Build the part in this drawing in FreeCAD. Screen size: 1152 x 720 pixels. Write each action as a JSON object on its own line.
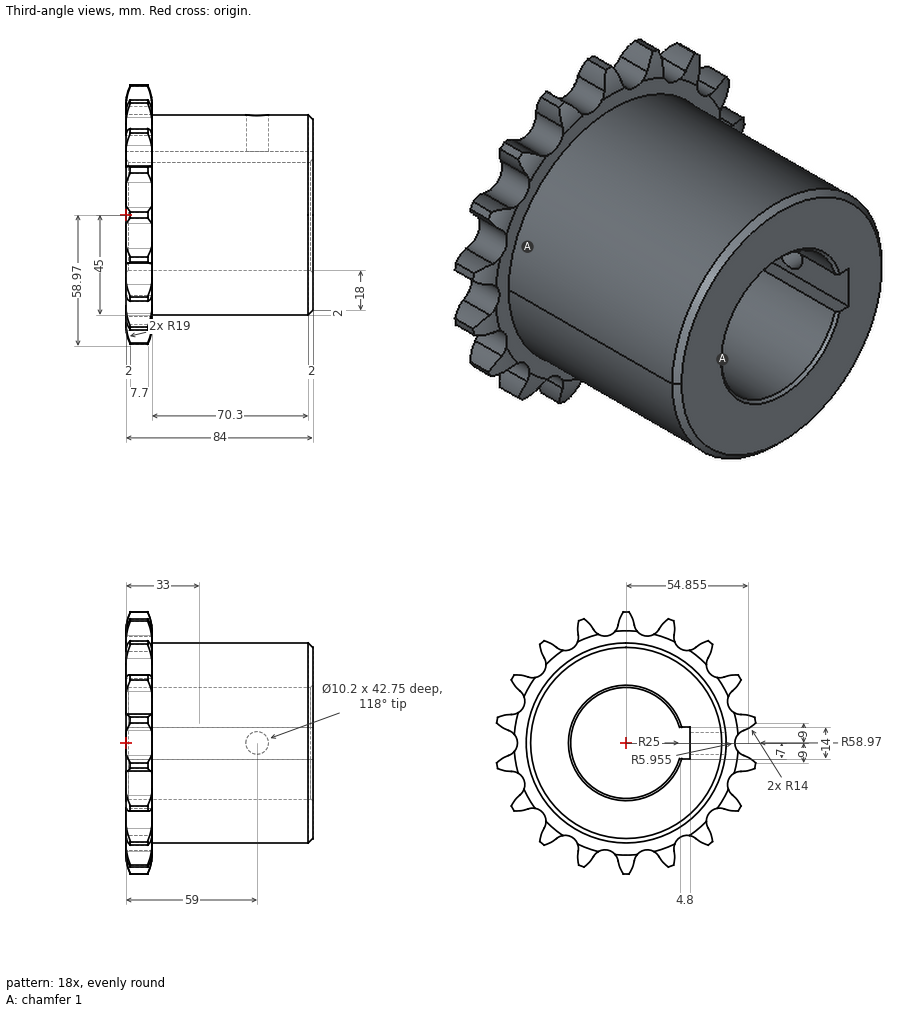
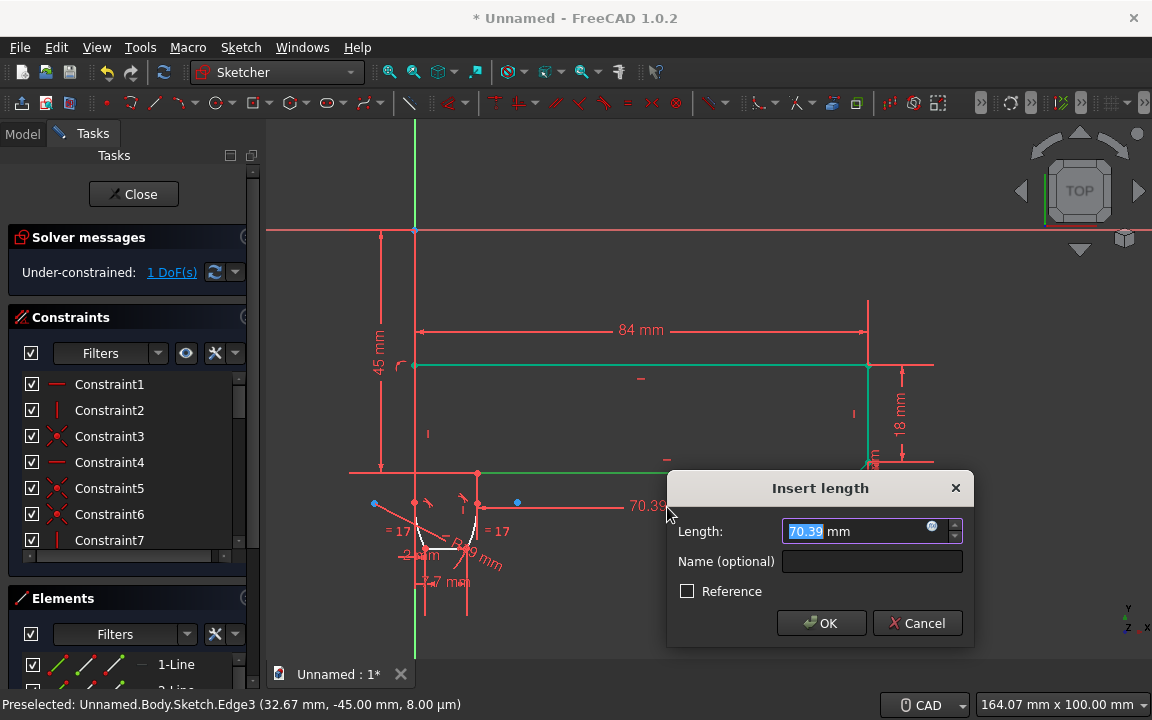
{"action": "type", "text": "70.3"}
{"action": "key", "text": "Return"}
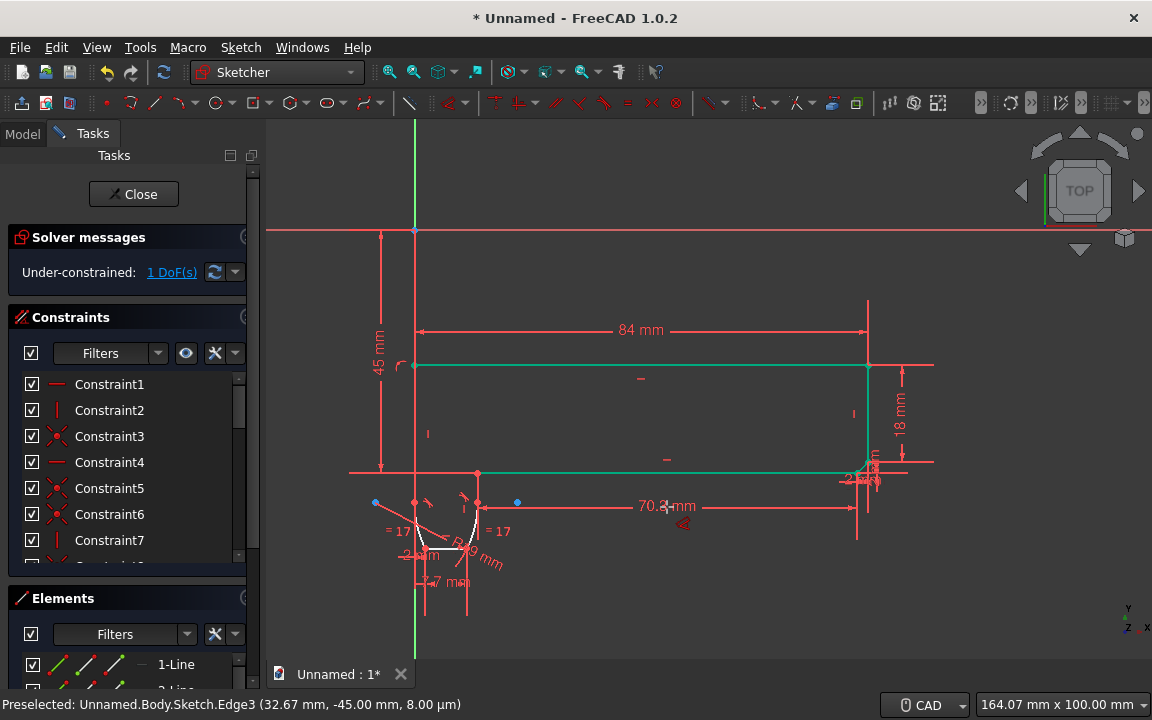
{"action": "left_click", "coordinate": [425, 549]}
{"action": "left_click", "coordinate": [381, 389]}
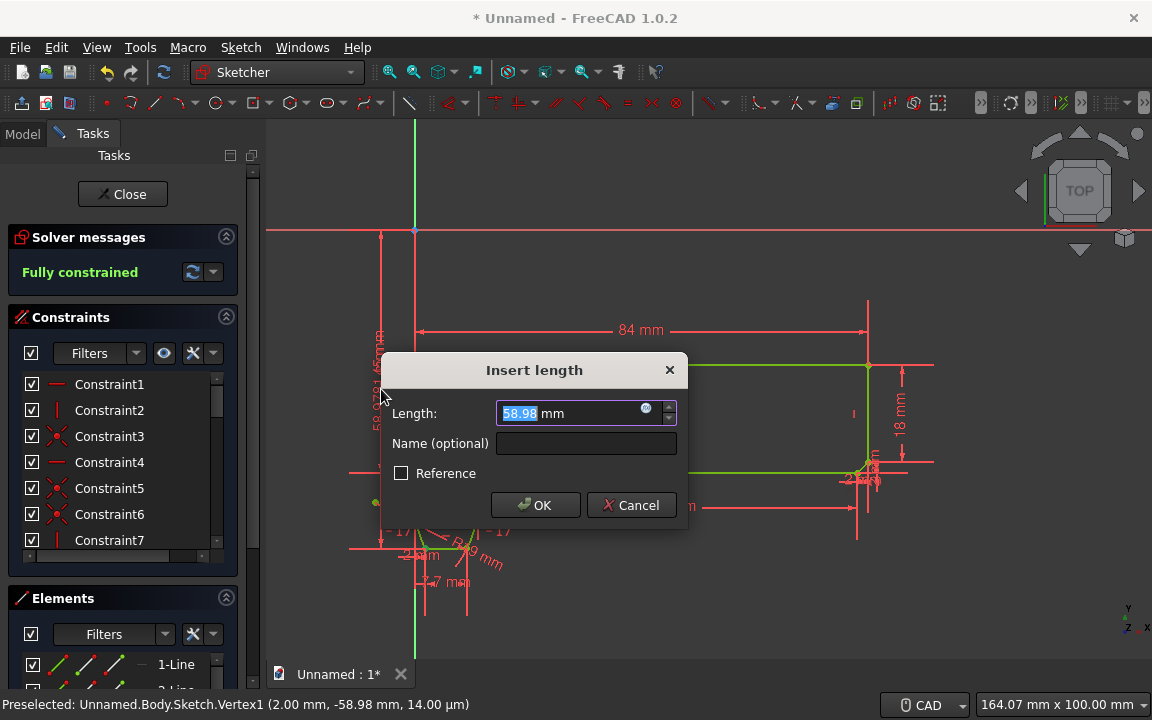
{"action": "type", "text": "58.97"}
{"action": "key", "text": "Return"}
{"action": "key", "text": "Escape"}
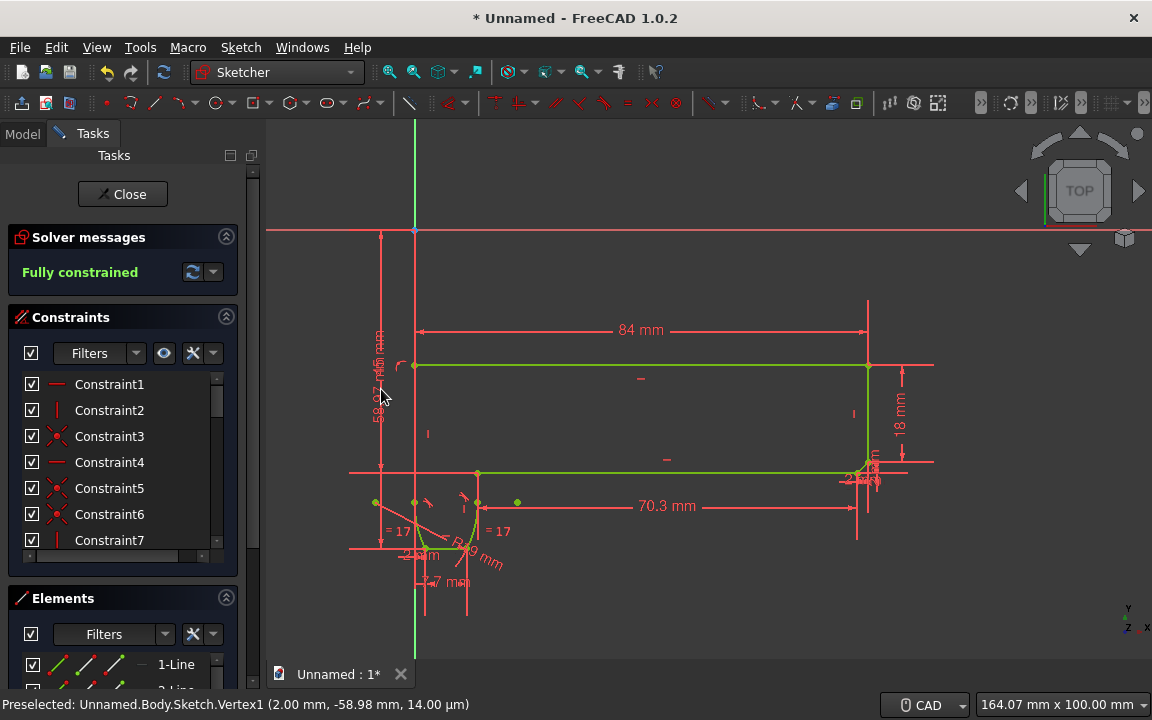
{"action": "left_click", "coordinate": [123, 194]}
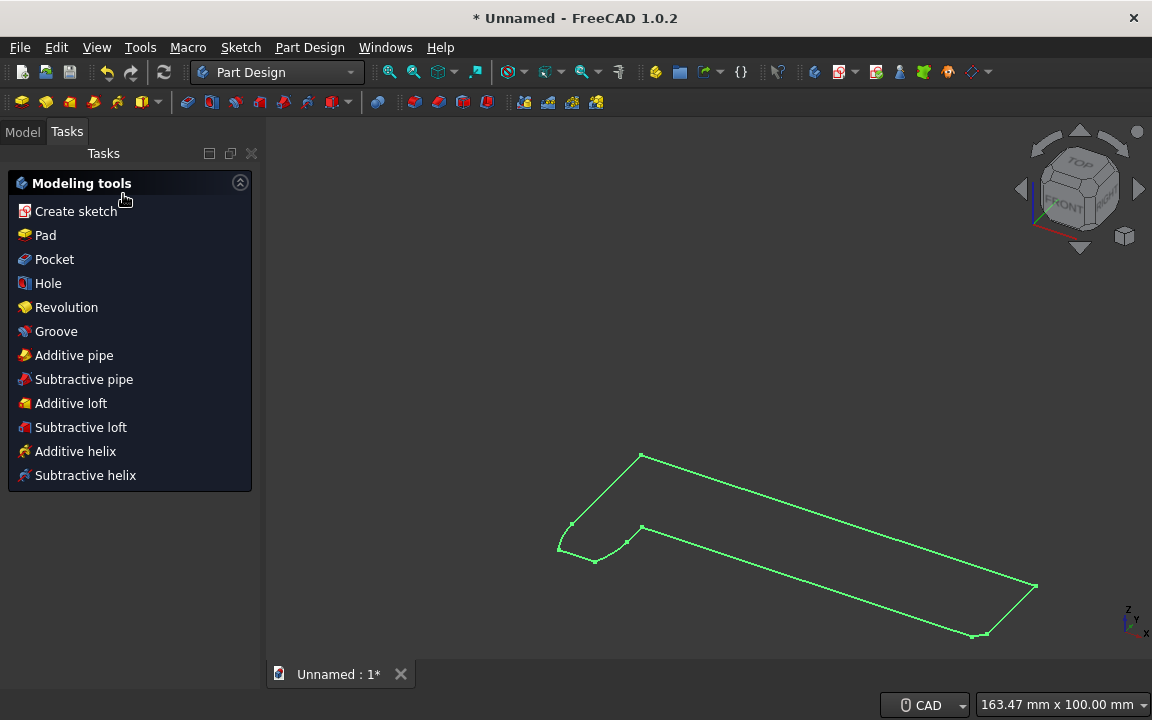
{"action": "left_click", "coordinate": [46, 102]}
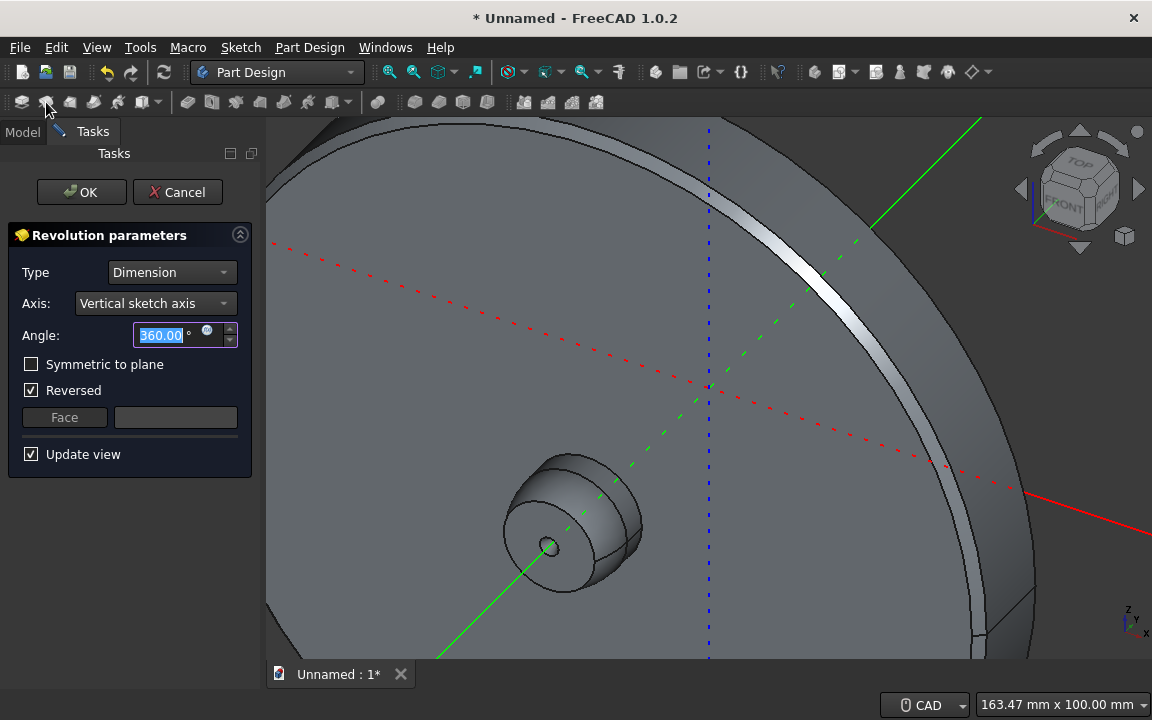
{"action": "left_click", "coordinate": [156, 304]}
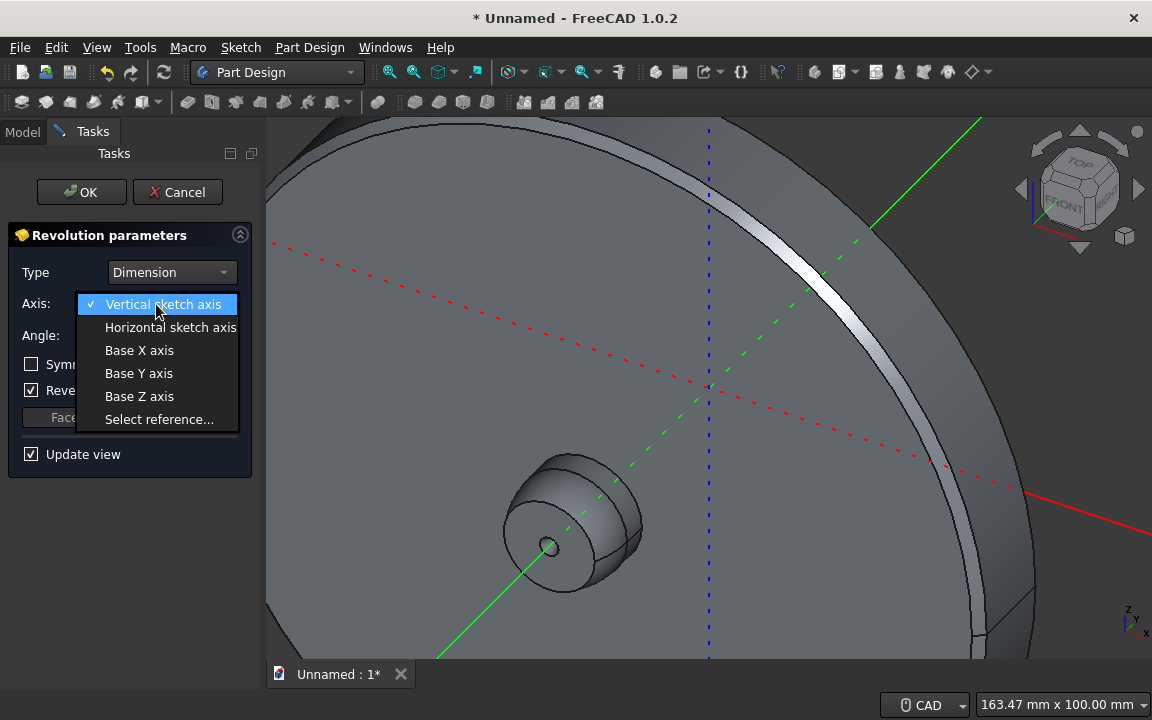
{"action": "left_click", "coordinate": [156, 328]}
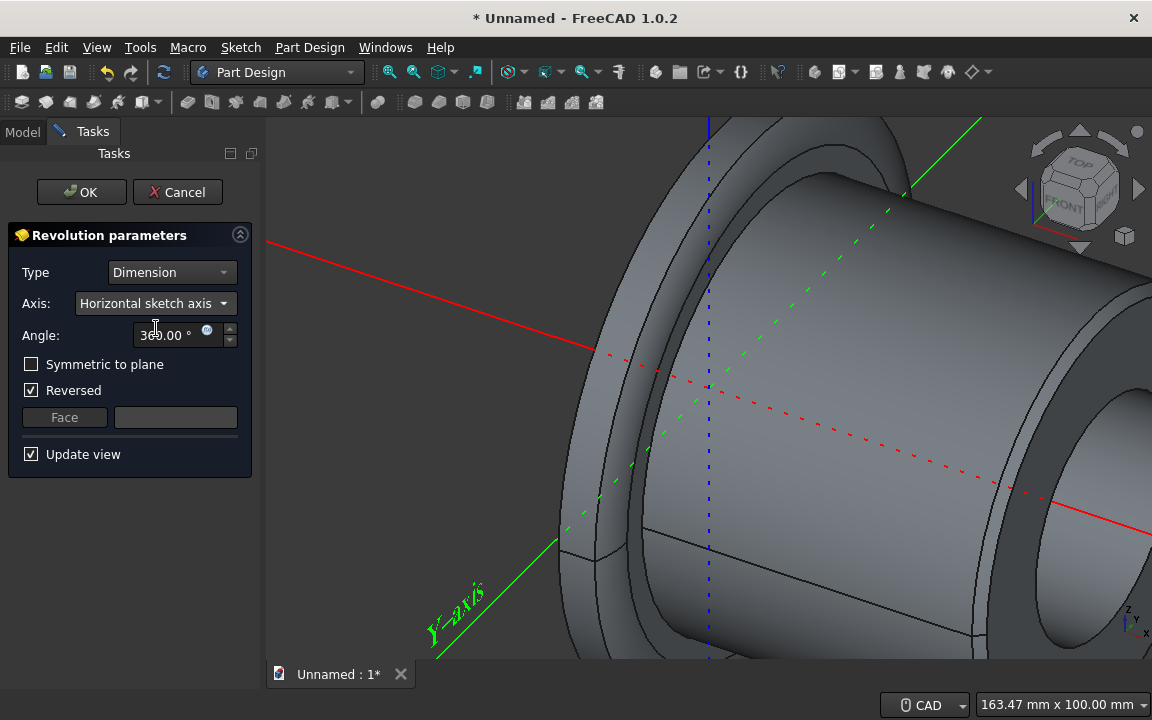
{"action": "left_click", "coordinate": [82, 192]}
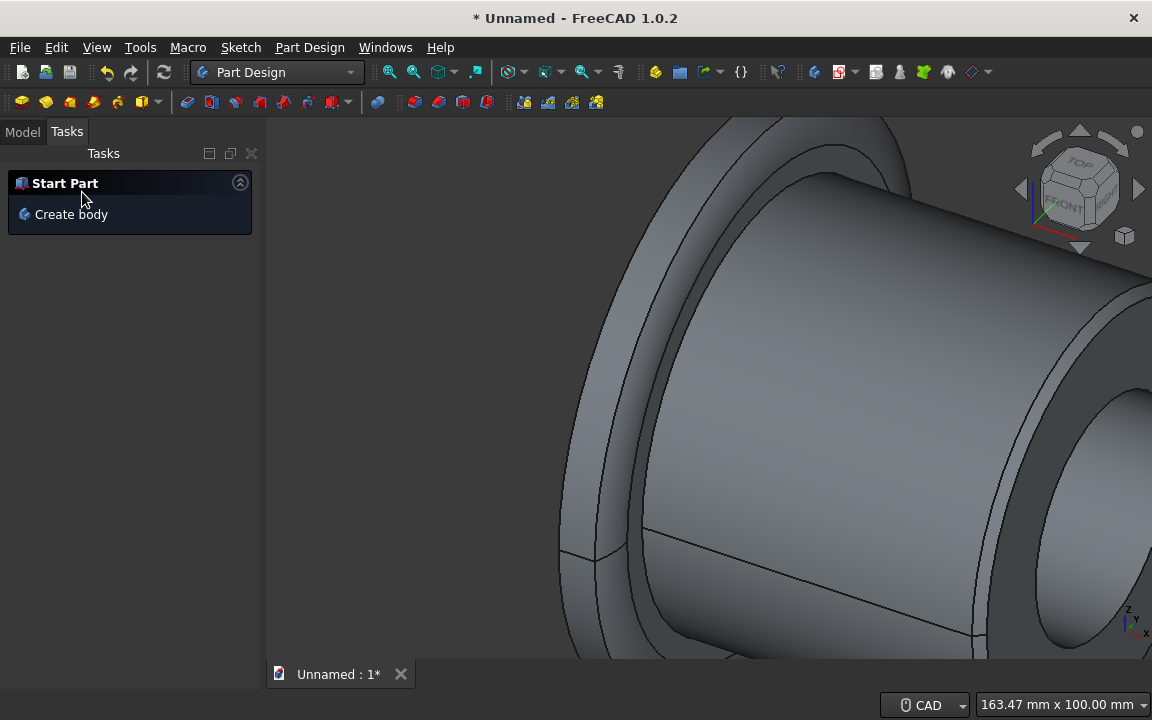
{"action": "left_click", "coordinate": [390, 72]}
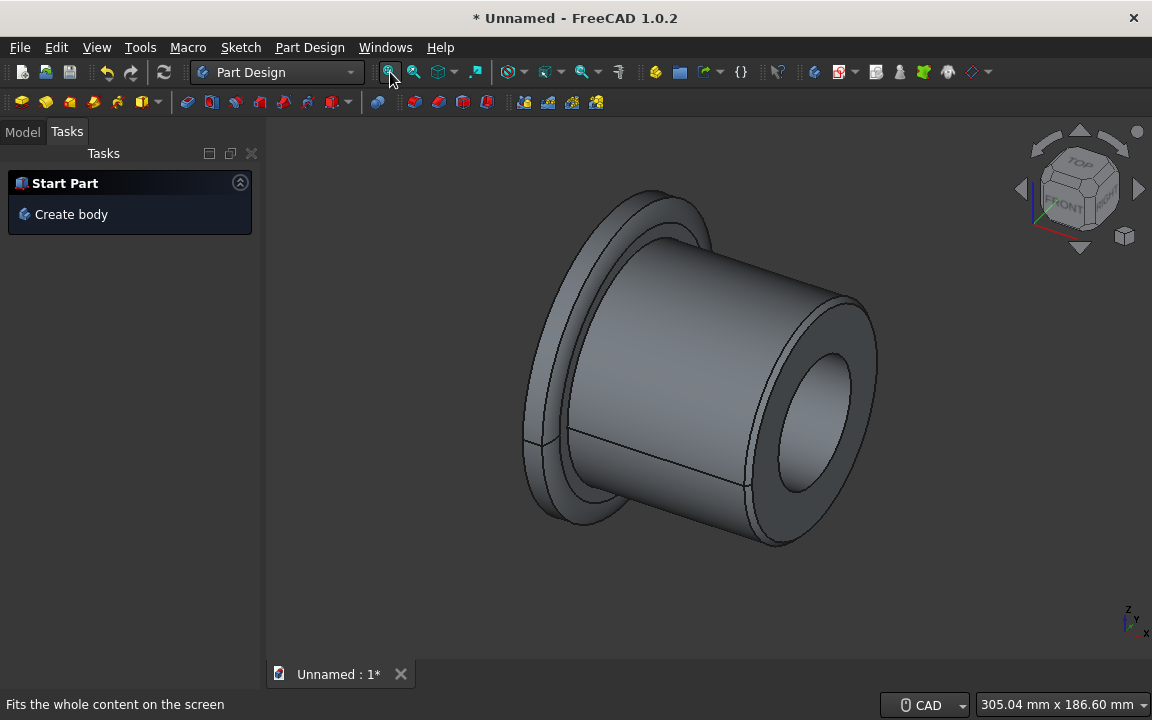
{"action": "left_click", "coordinate": [850, 445]}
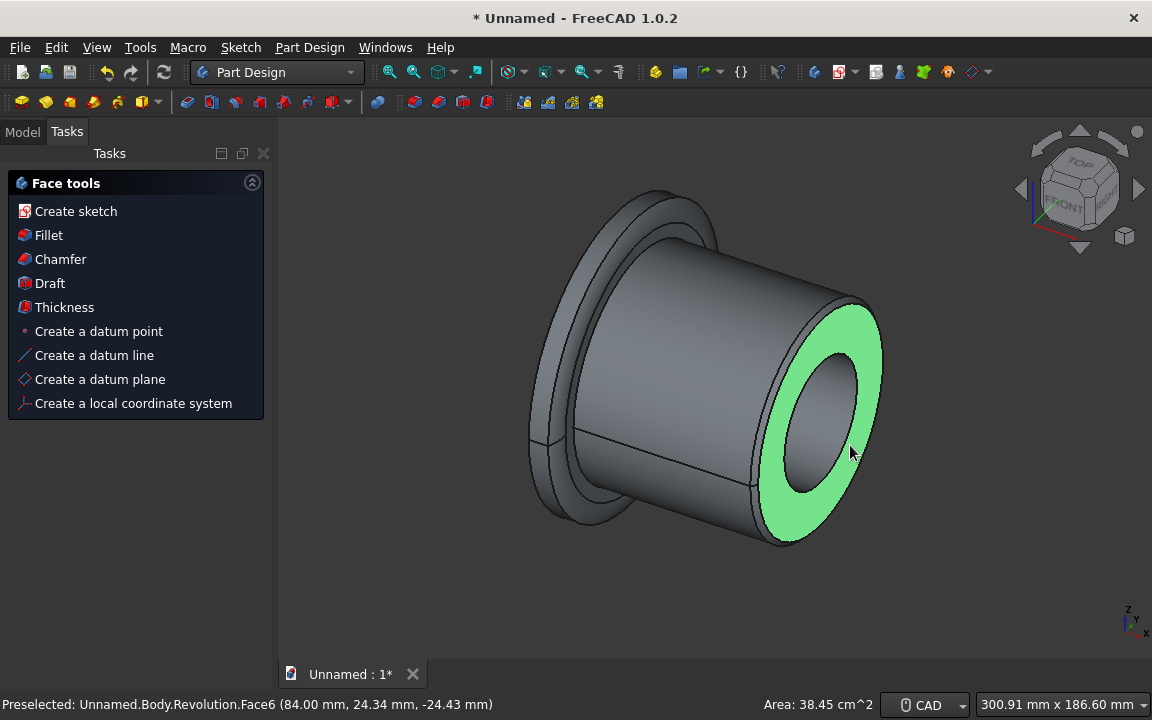
{"action": "left_click", "coordinate": [840, 72]}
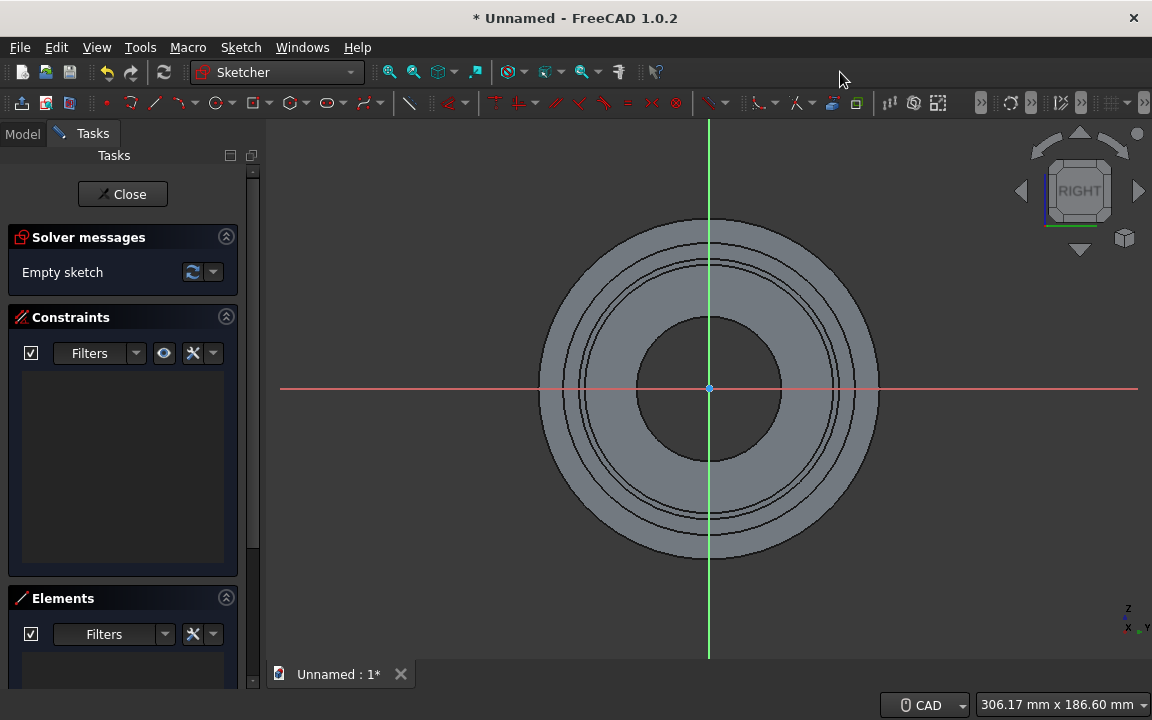
{"action": "scroll", "coordinate": [772, 389], "scroll_direction": "up", "scroll_amount": 9}